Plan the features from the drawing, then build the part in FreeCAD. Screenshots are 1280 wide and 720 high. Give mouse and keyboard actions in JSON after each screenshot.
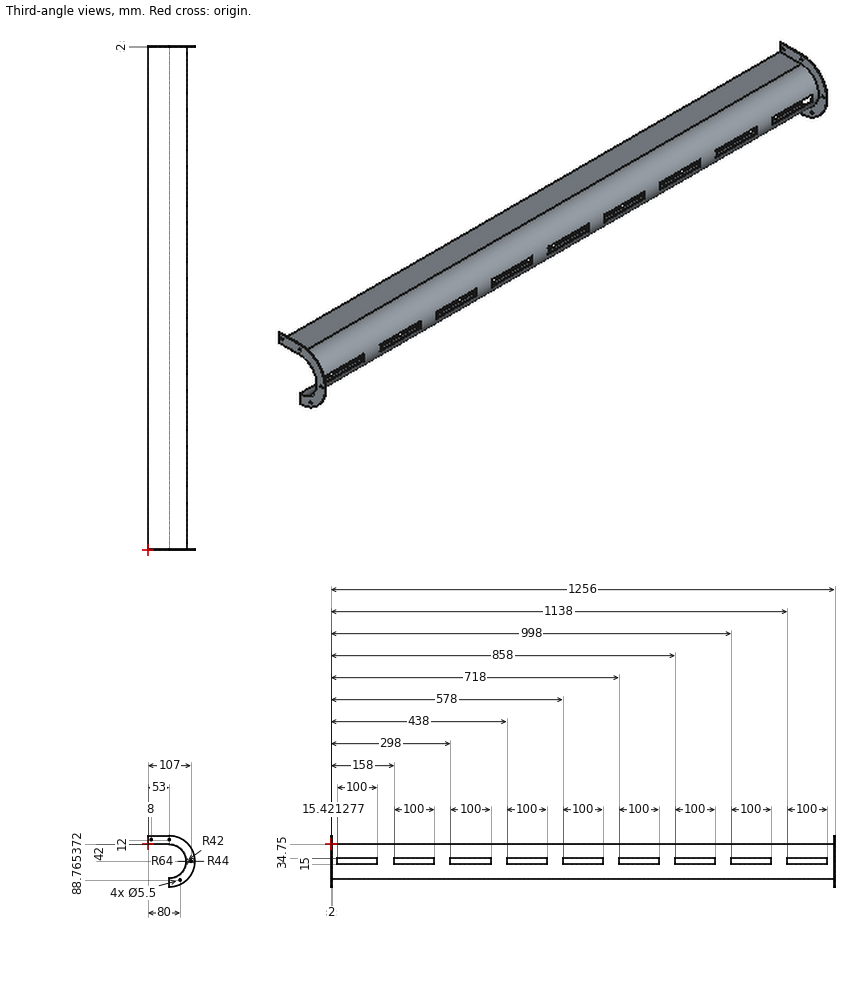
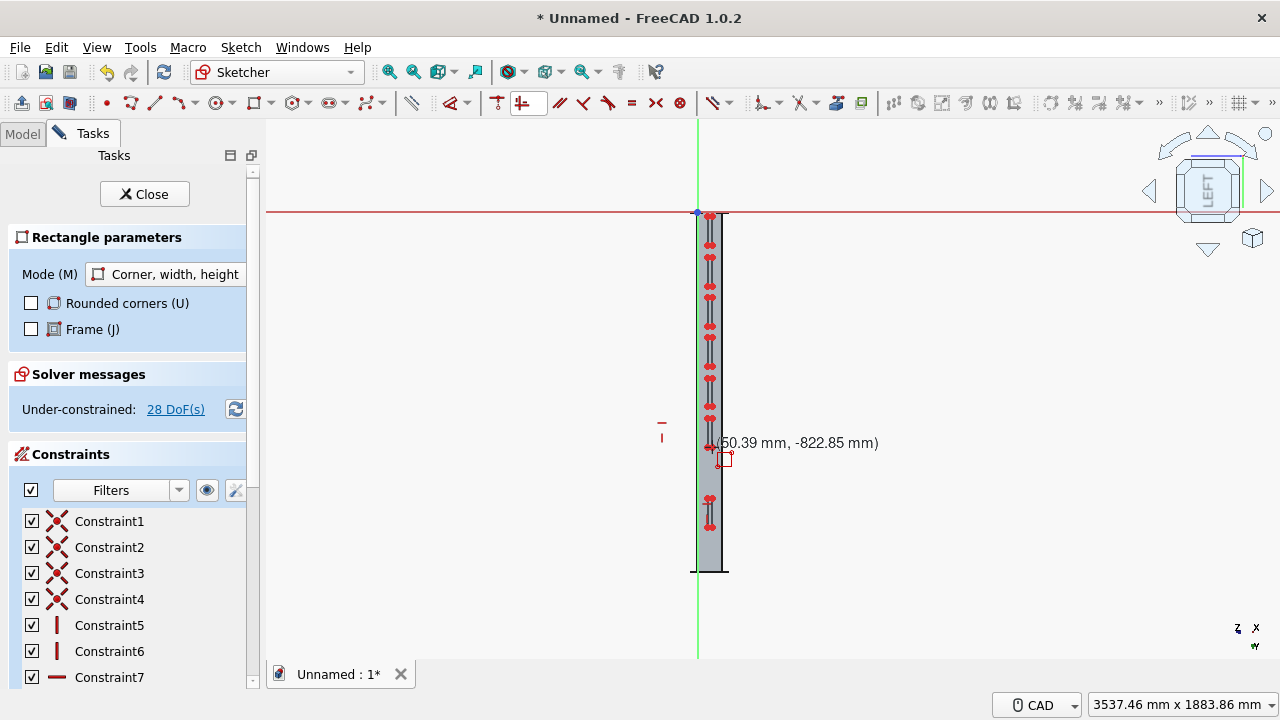
{"action": "scroll", "coordinate": [708, 458], "scroll_direction": "up", "scroll_amount": 7}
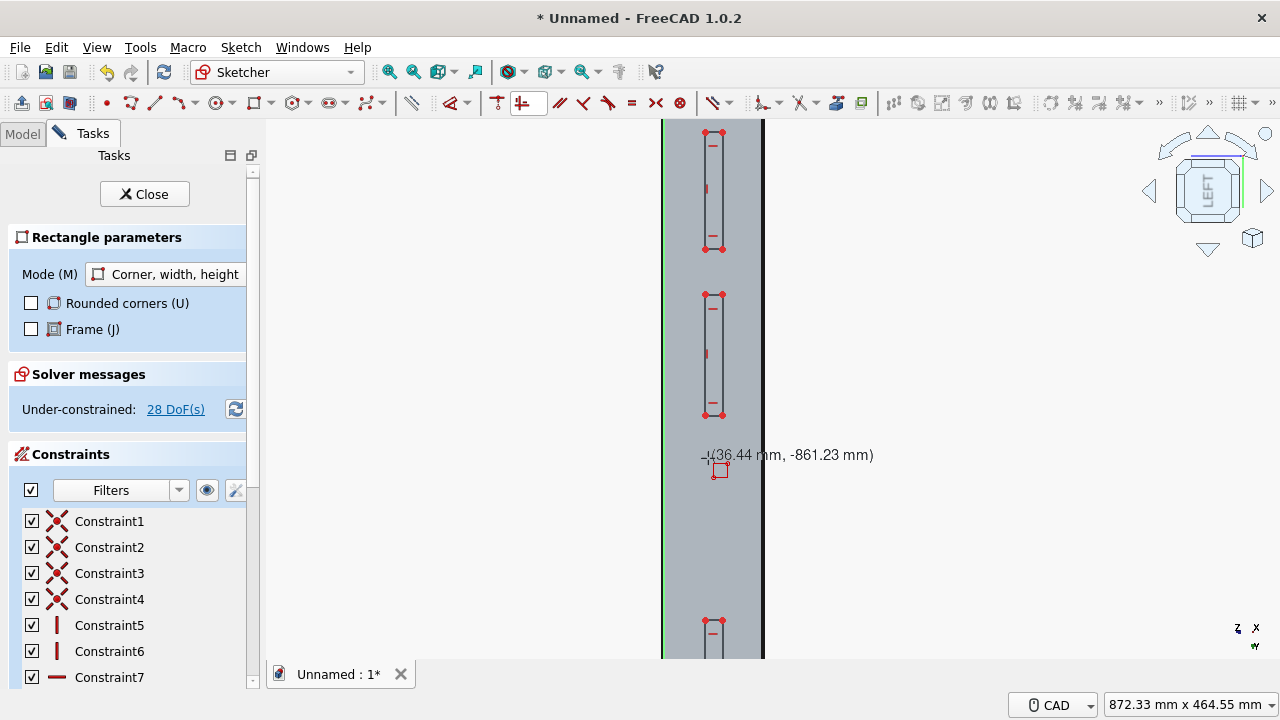
{"action": "left_click", "coordinate": [705, 456]}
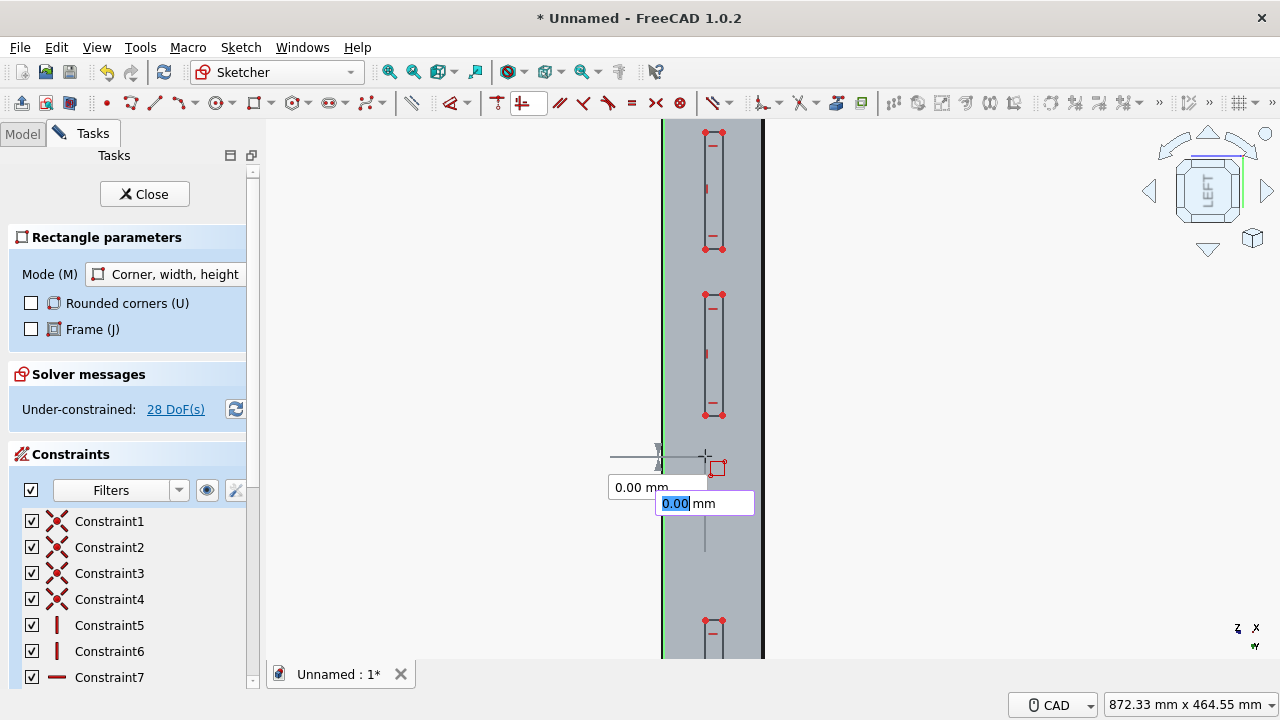
{"action": "scroll", "coordinate": [708, 458], "scroll_direction": "down", "scroll_amount": 7}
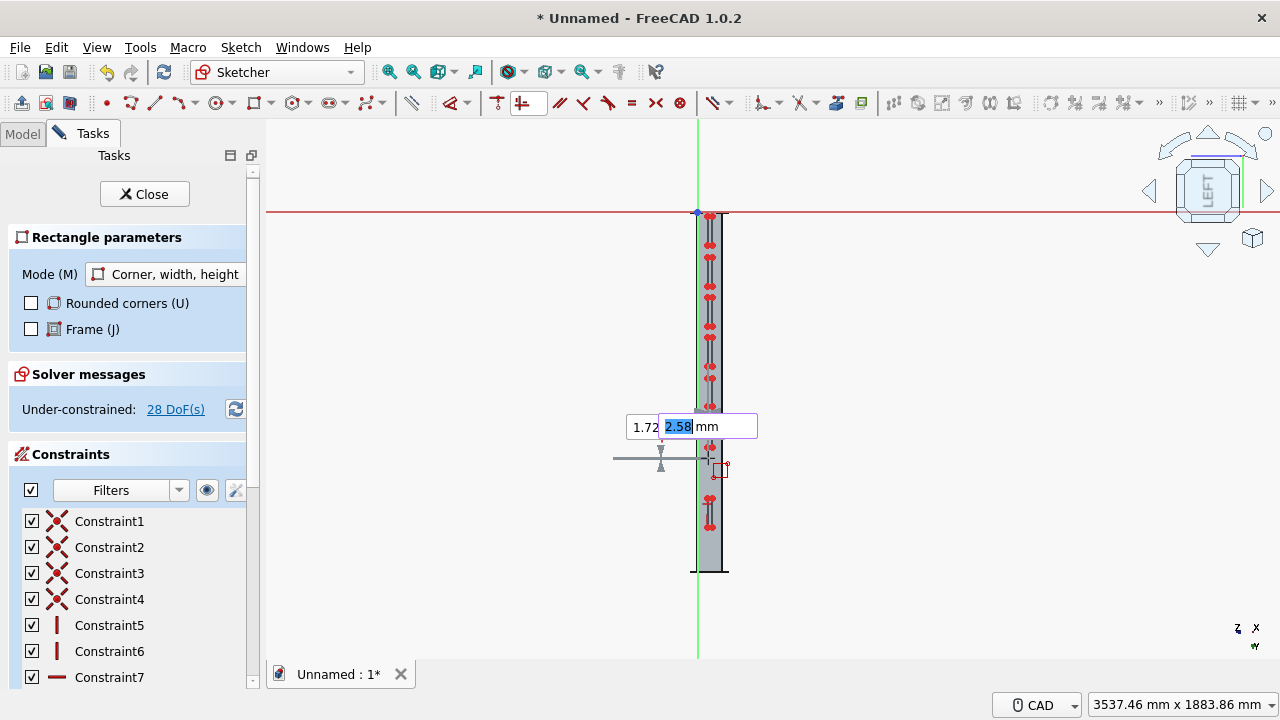
{"action": "scroll", "coordinate": [712, 487], "scroll_direction": "up", "scroll_amount": 2}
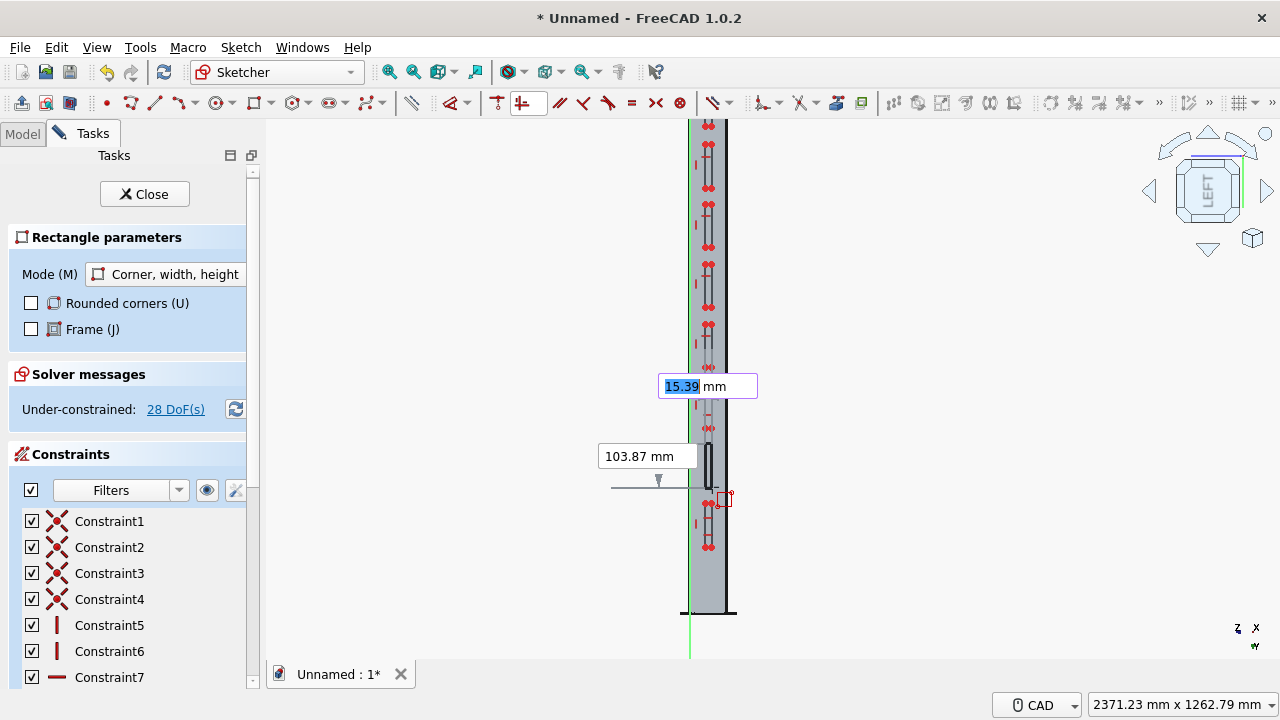
{"action": "left_click", "coordinate": [712, 486]}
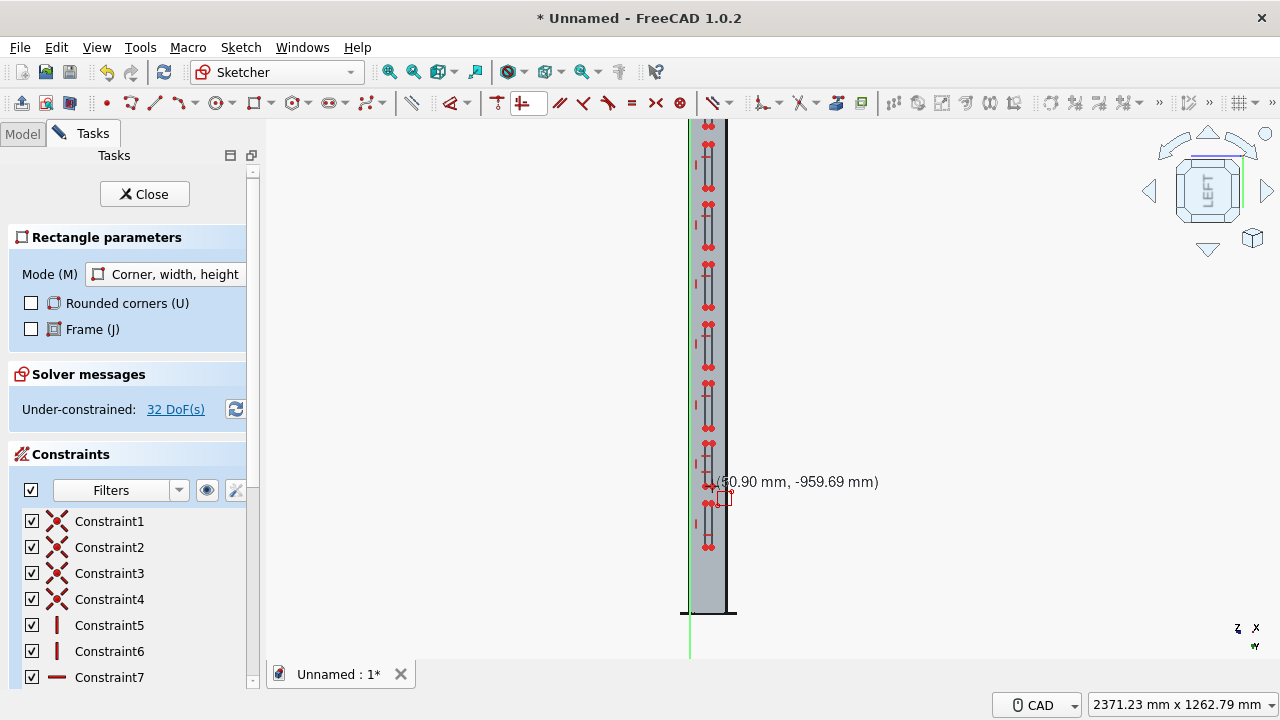
{"action": "scroll", "coordinate": [705, 563], "scroll_direction": "up", "scroll_amount": 5}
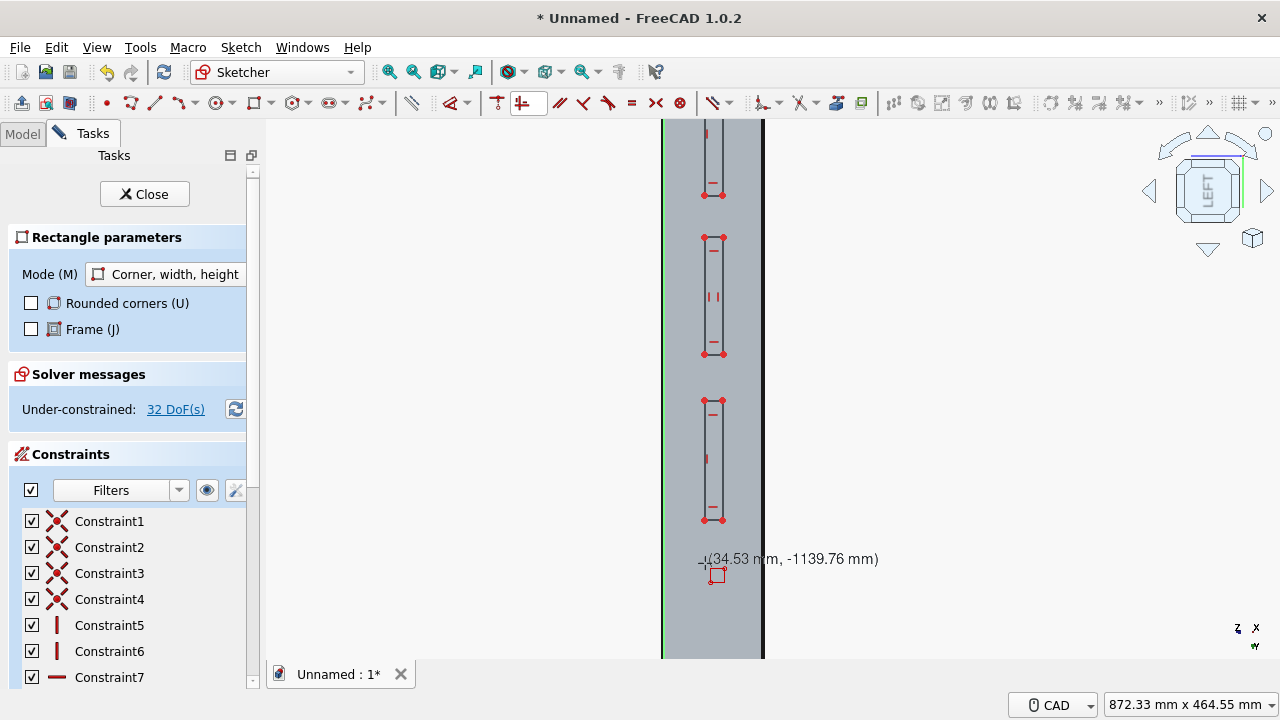
{"action": "left_click", "coordinate": [705, 562]}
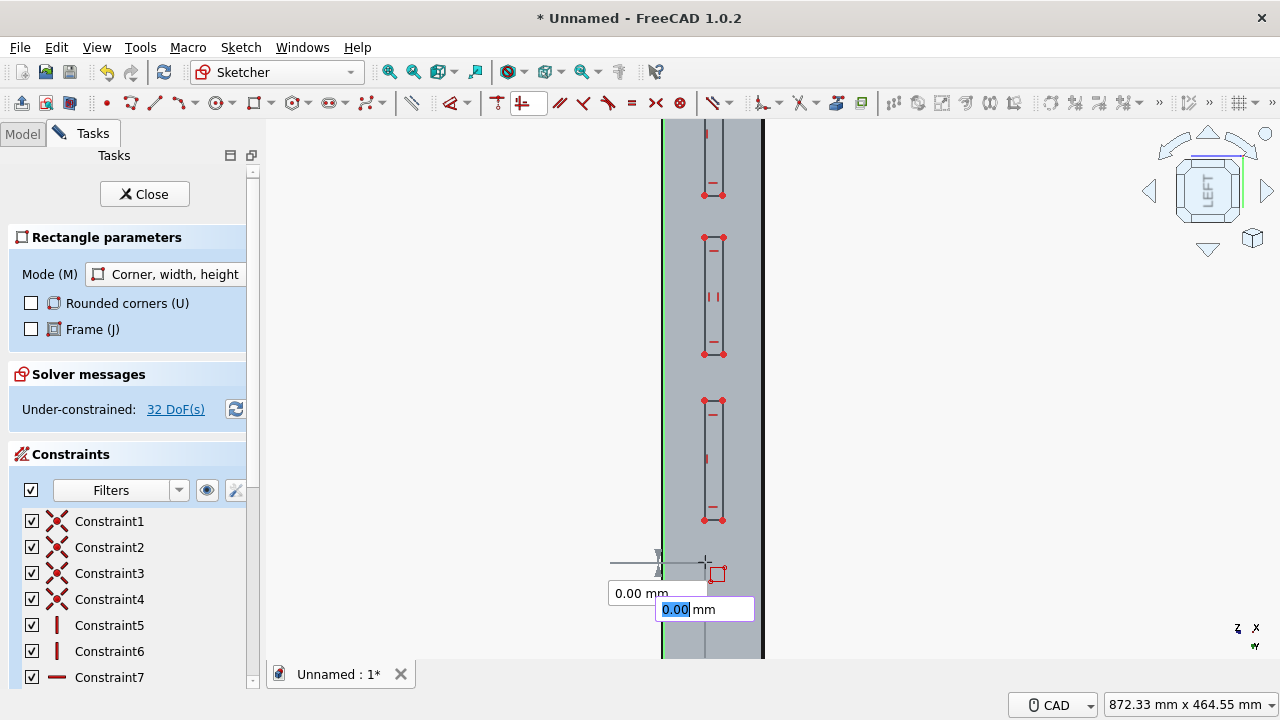
{"action": "scroll", "coordinate": [708, 530], "scroll_direction": "down", "scroll_amount": 7}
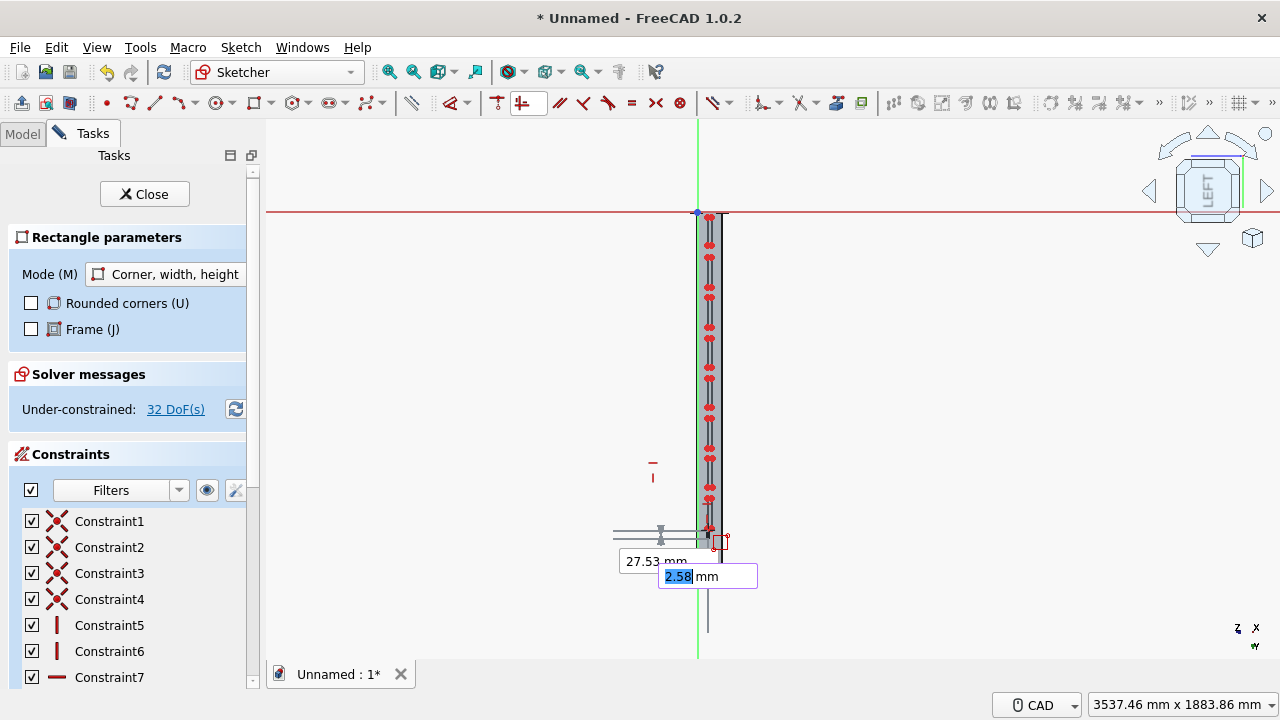
{"action": "left_click", "coordinate": [712, 567]}
{"action": "key", "text": "Escape"}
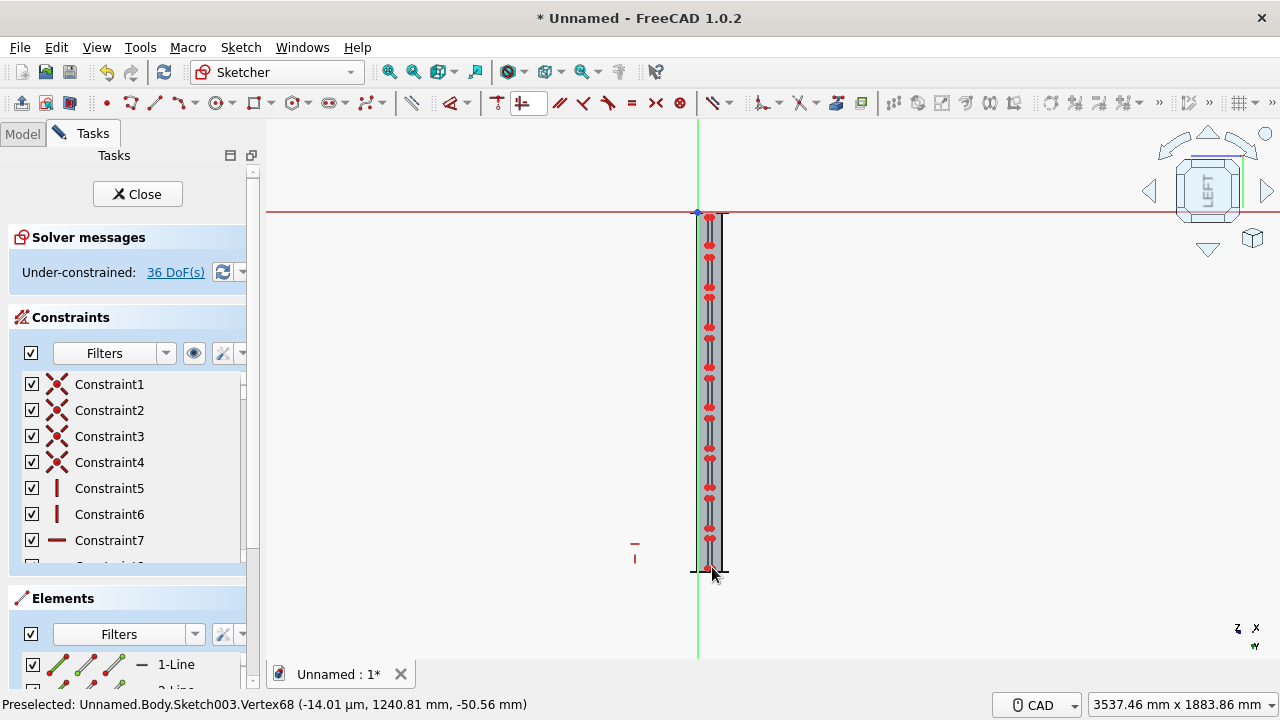
{"action": "left_click", "coordinate": [450, 104]}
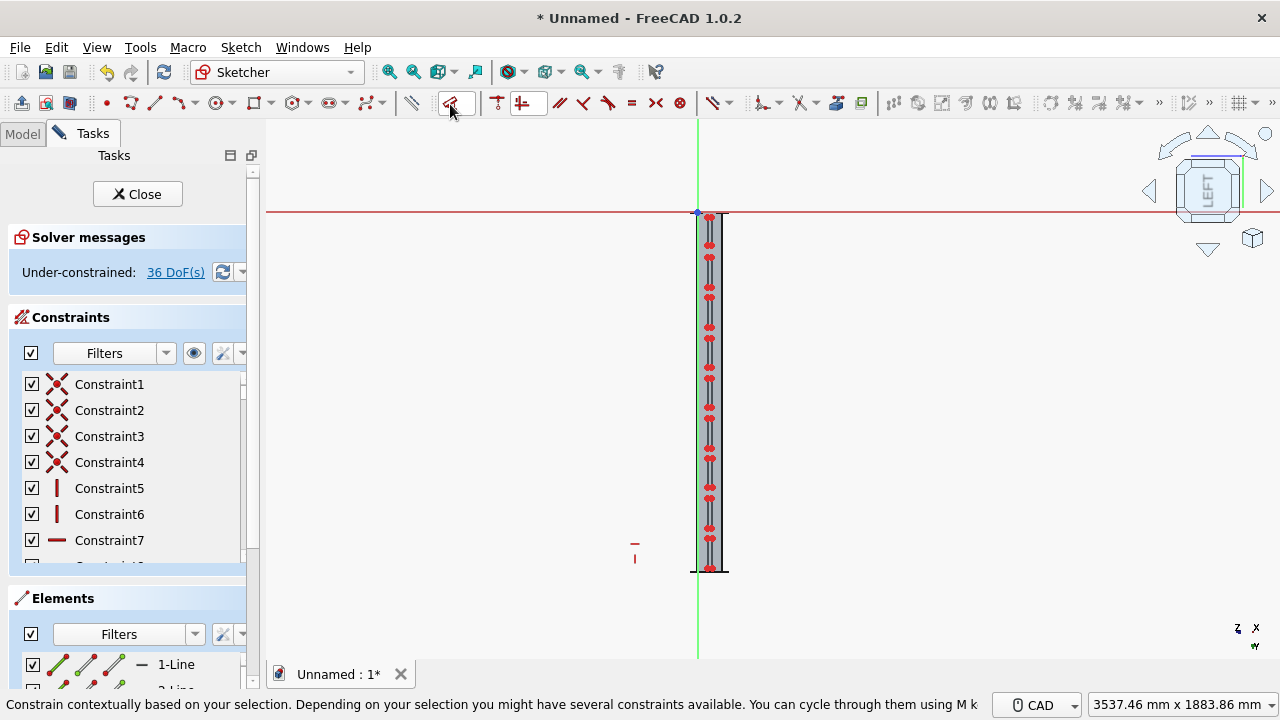
{"action": "scroll", "coordinate": [710, 246], "scroll_direction": "up", "scroll_amount": 12}